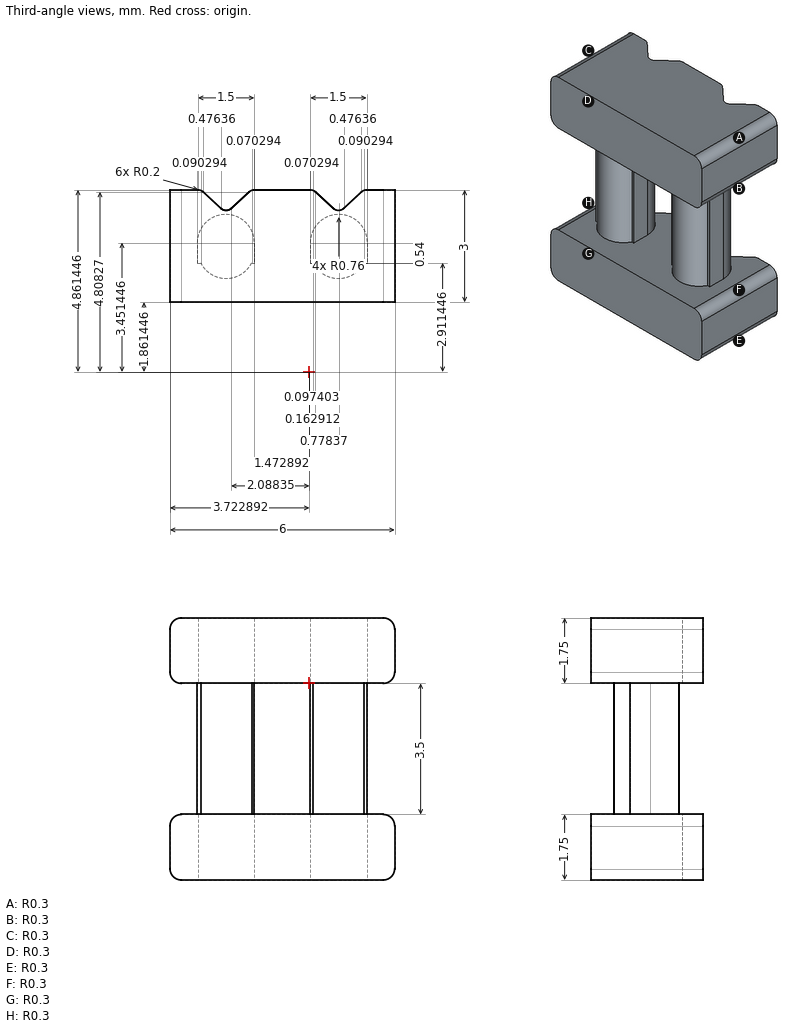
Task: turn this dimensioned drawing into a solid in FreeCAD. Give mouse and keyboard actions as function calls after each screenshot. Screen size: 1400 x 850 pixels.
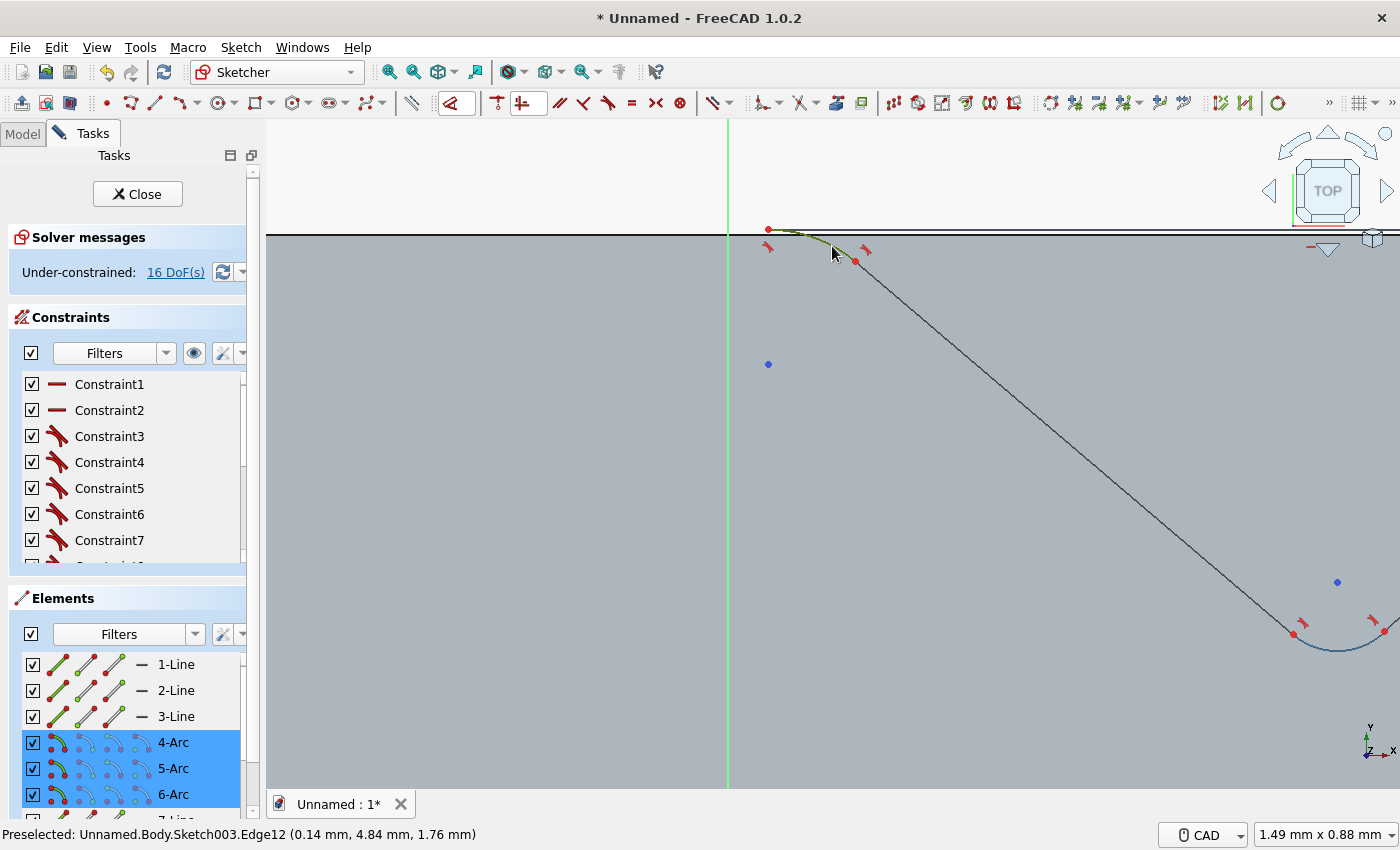
click(632, 104)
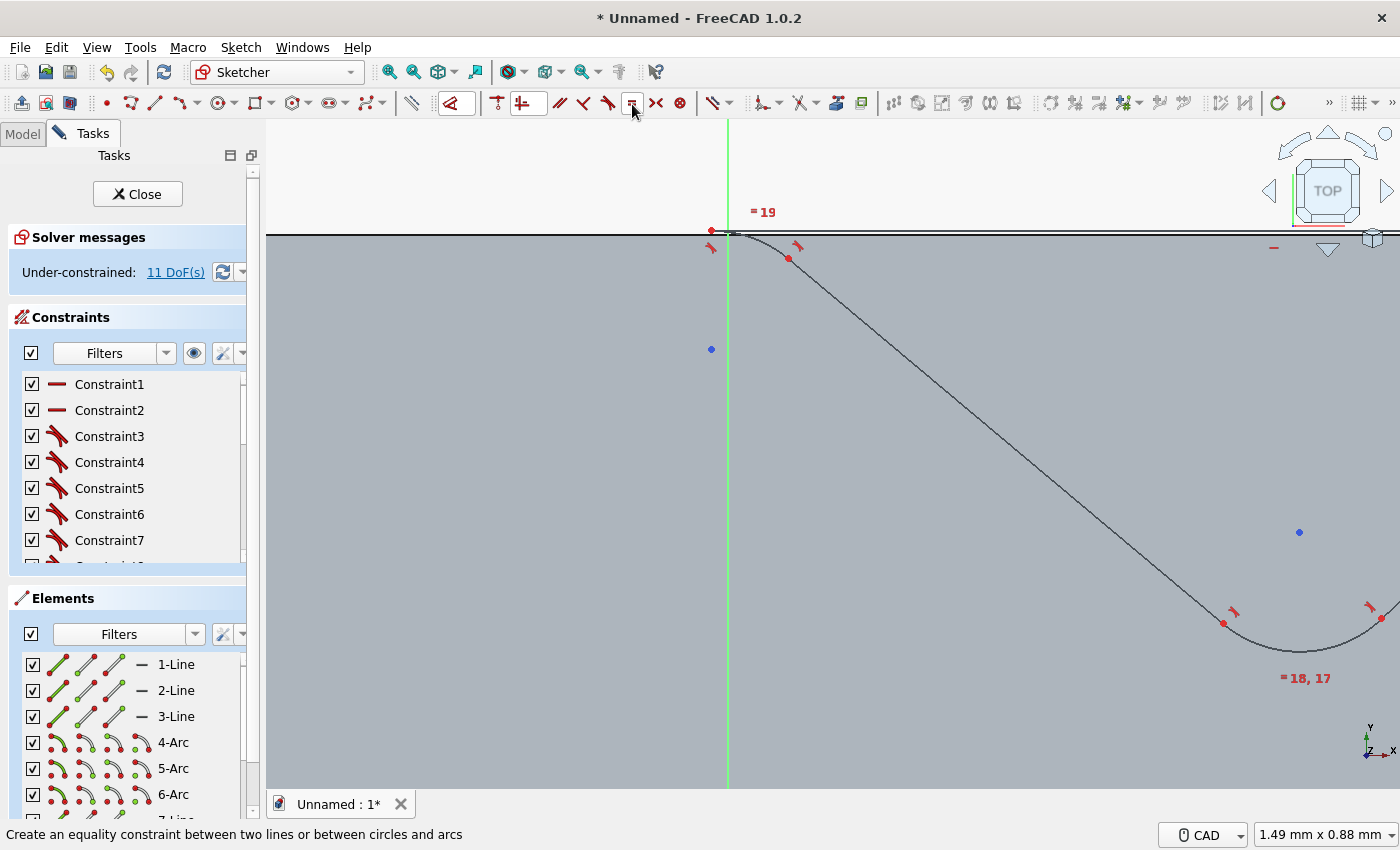
scroll(838, 251, down, 11)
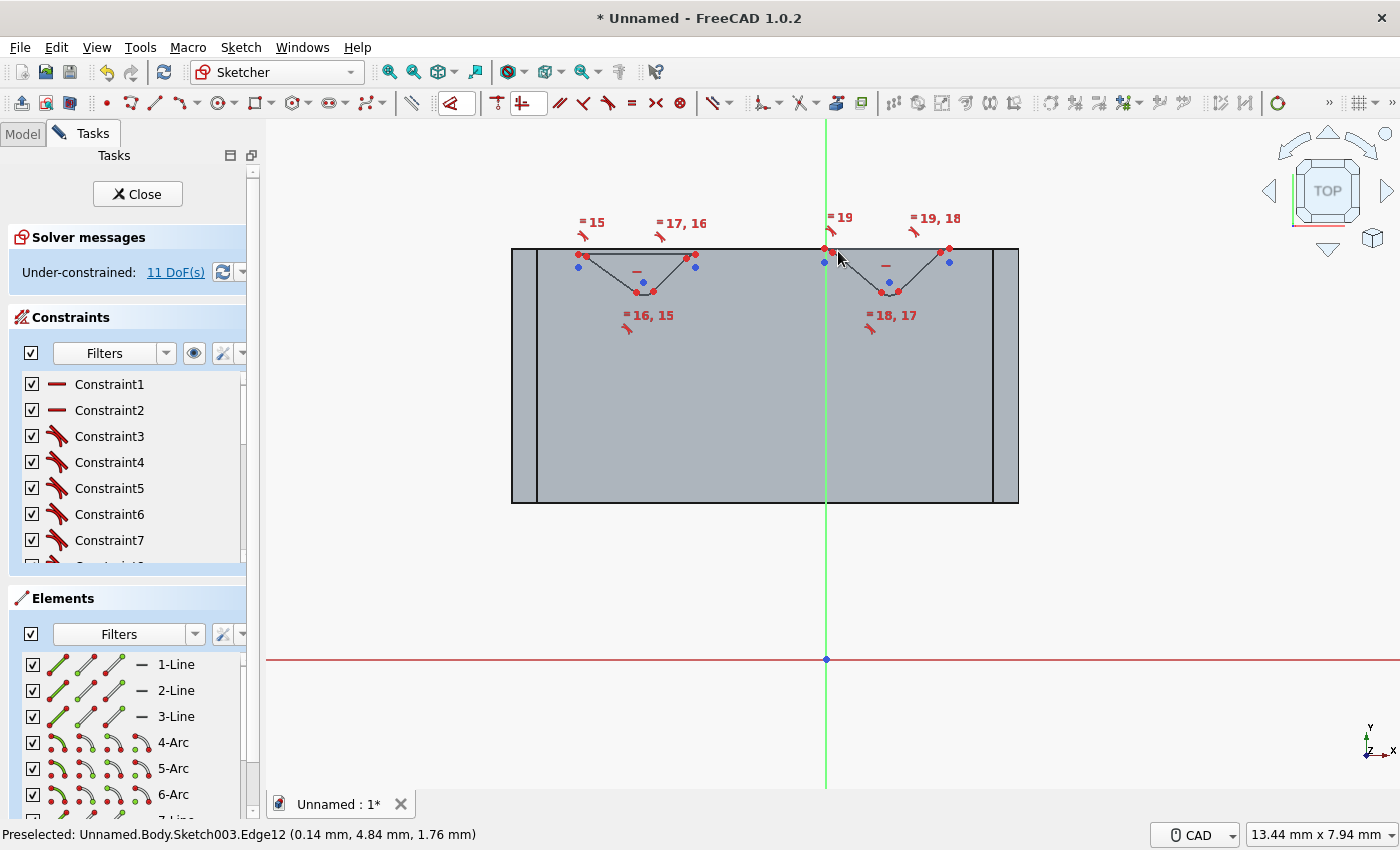
scroll(584, 256, up, 13)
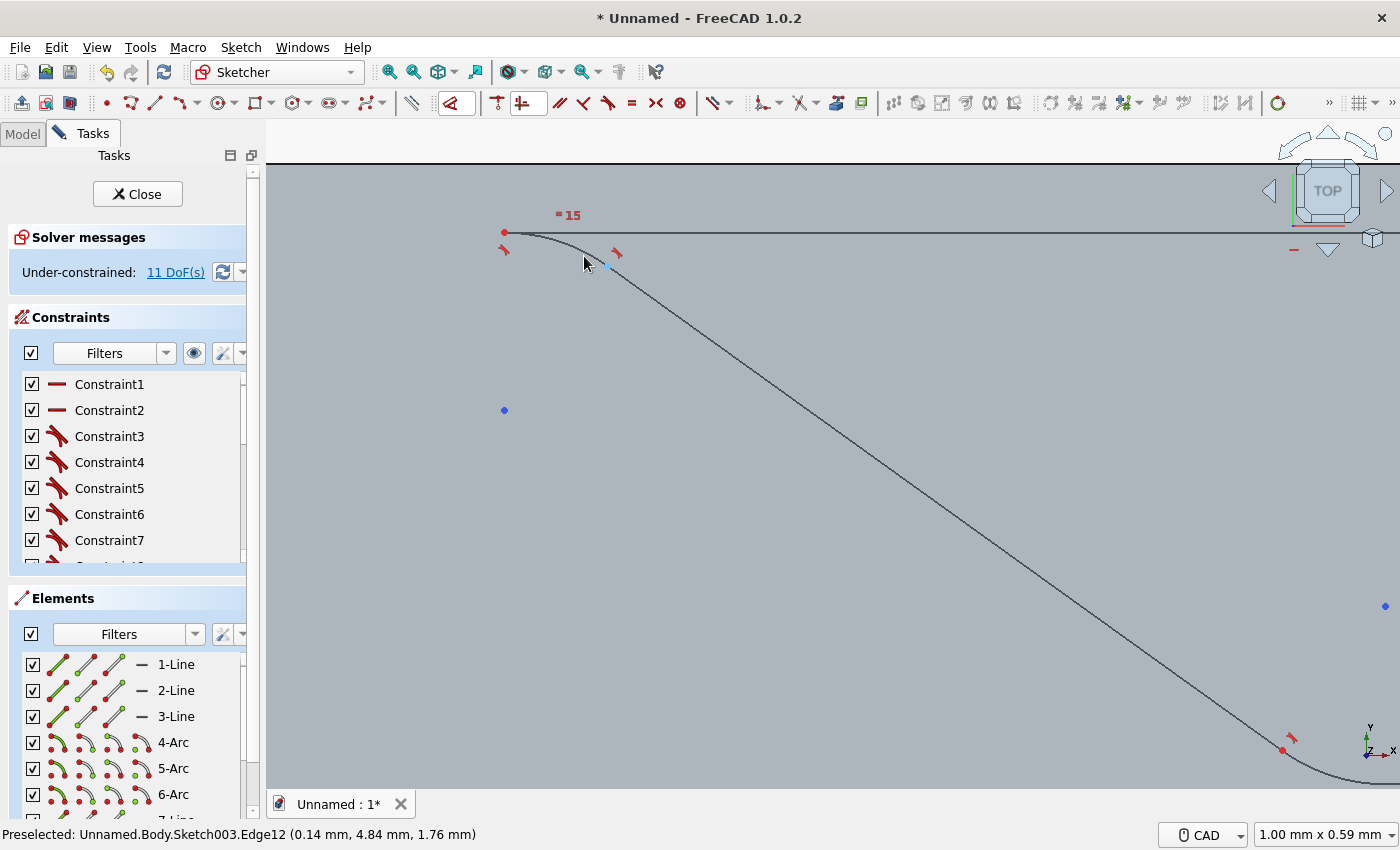
click(579, 249)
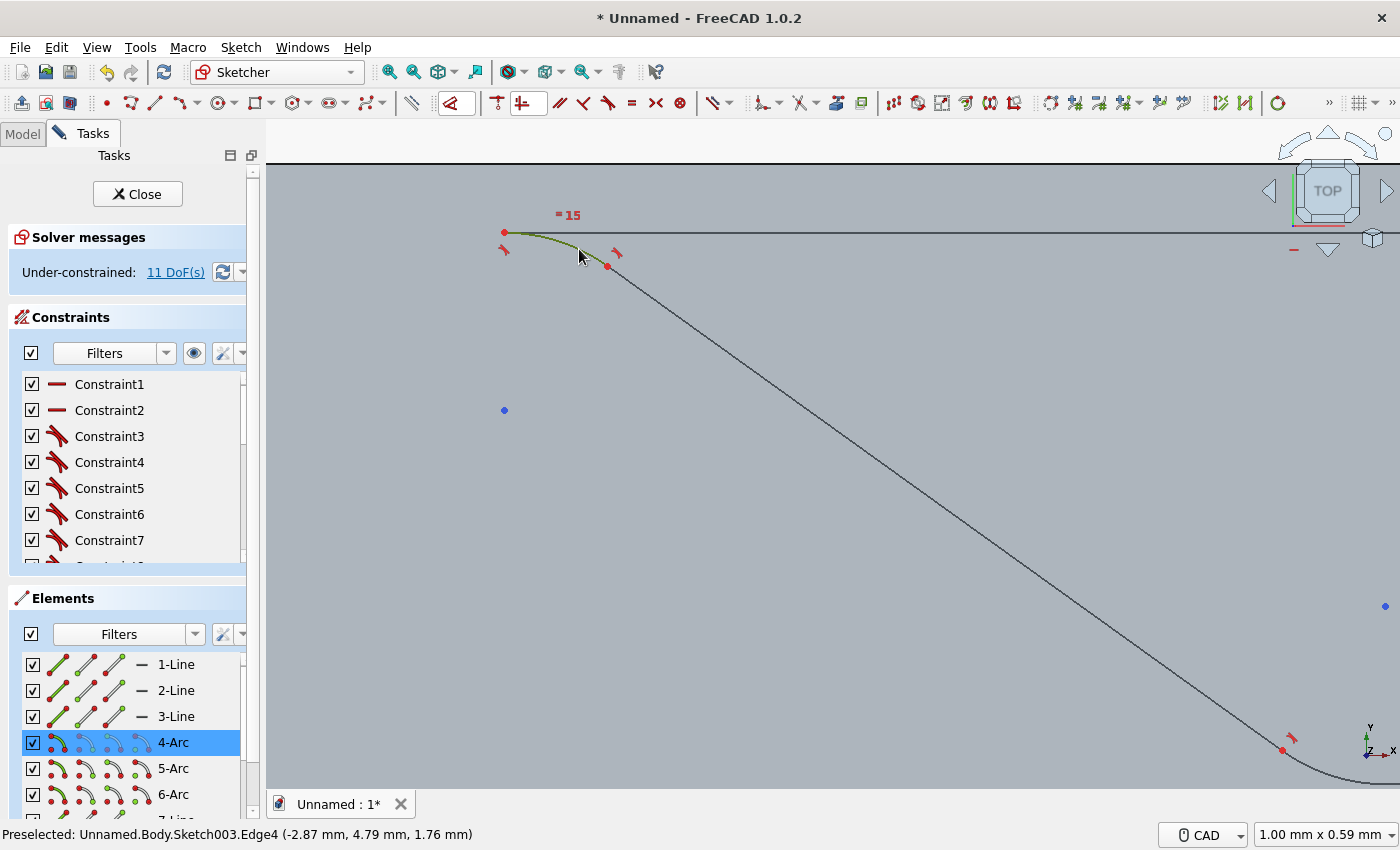
click(470, 104)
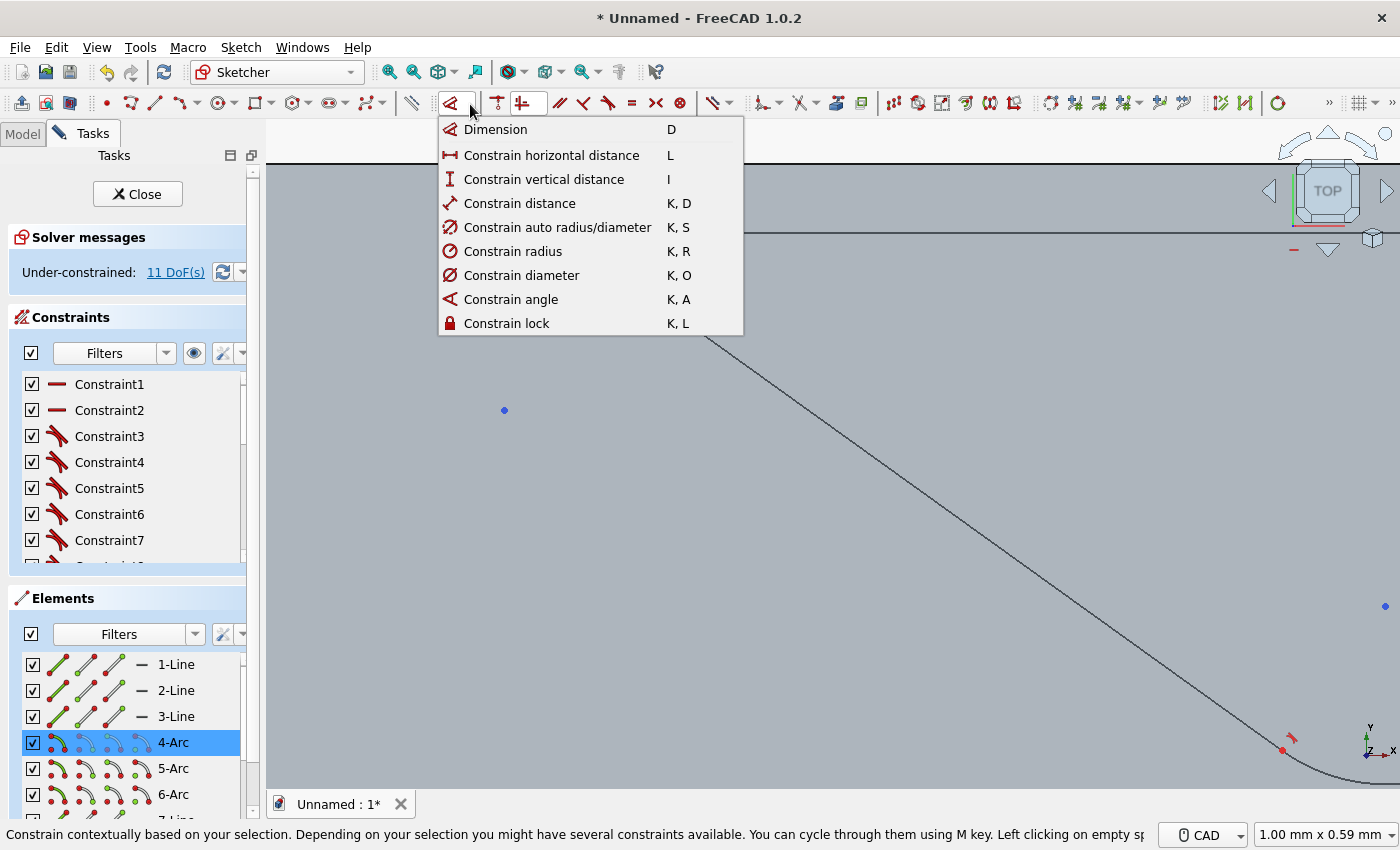
click(591, 251)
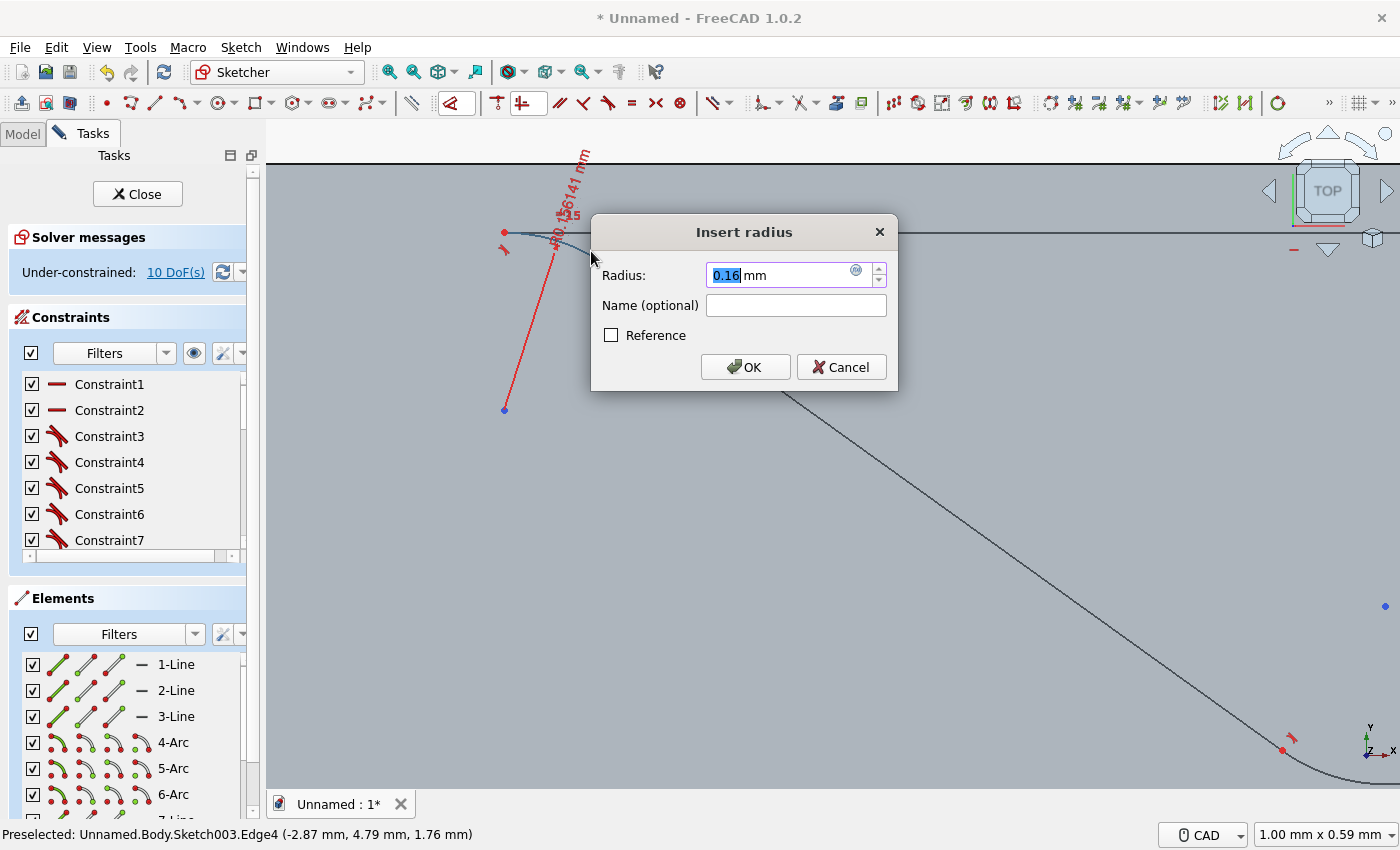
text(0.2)
key(Return)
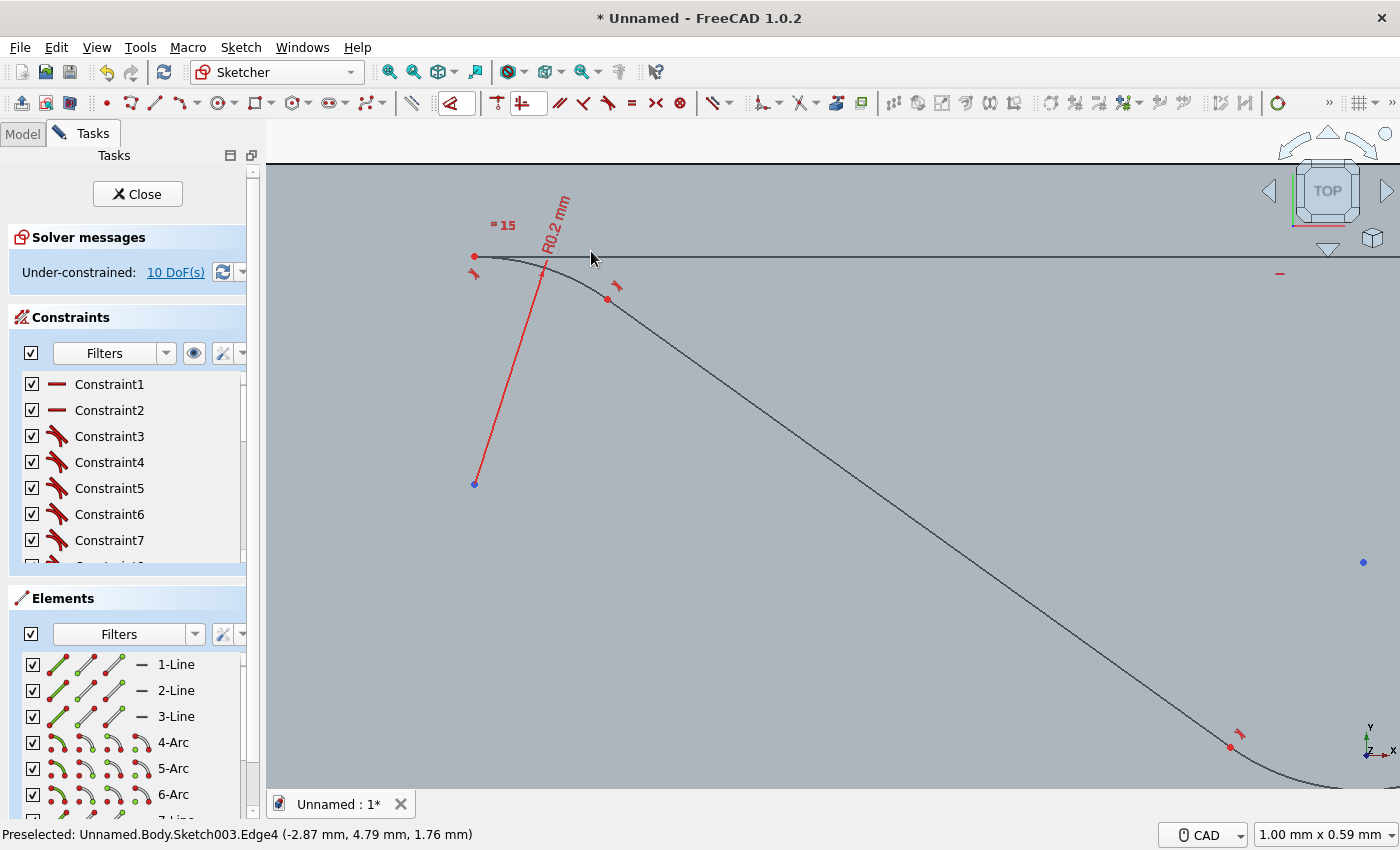
scroll(584, 256, down, 13)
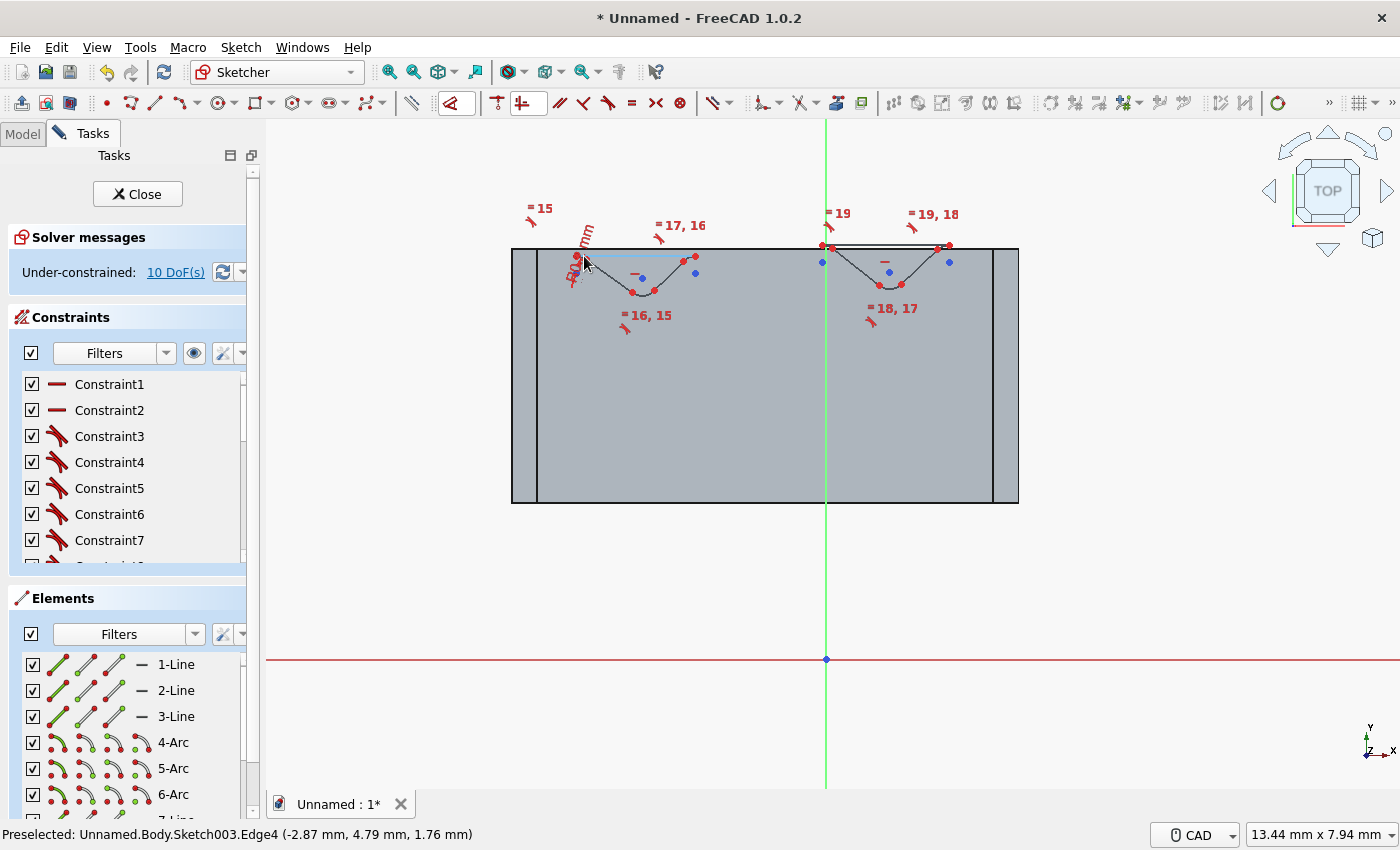
click(612, 256)